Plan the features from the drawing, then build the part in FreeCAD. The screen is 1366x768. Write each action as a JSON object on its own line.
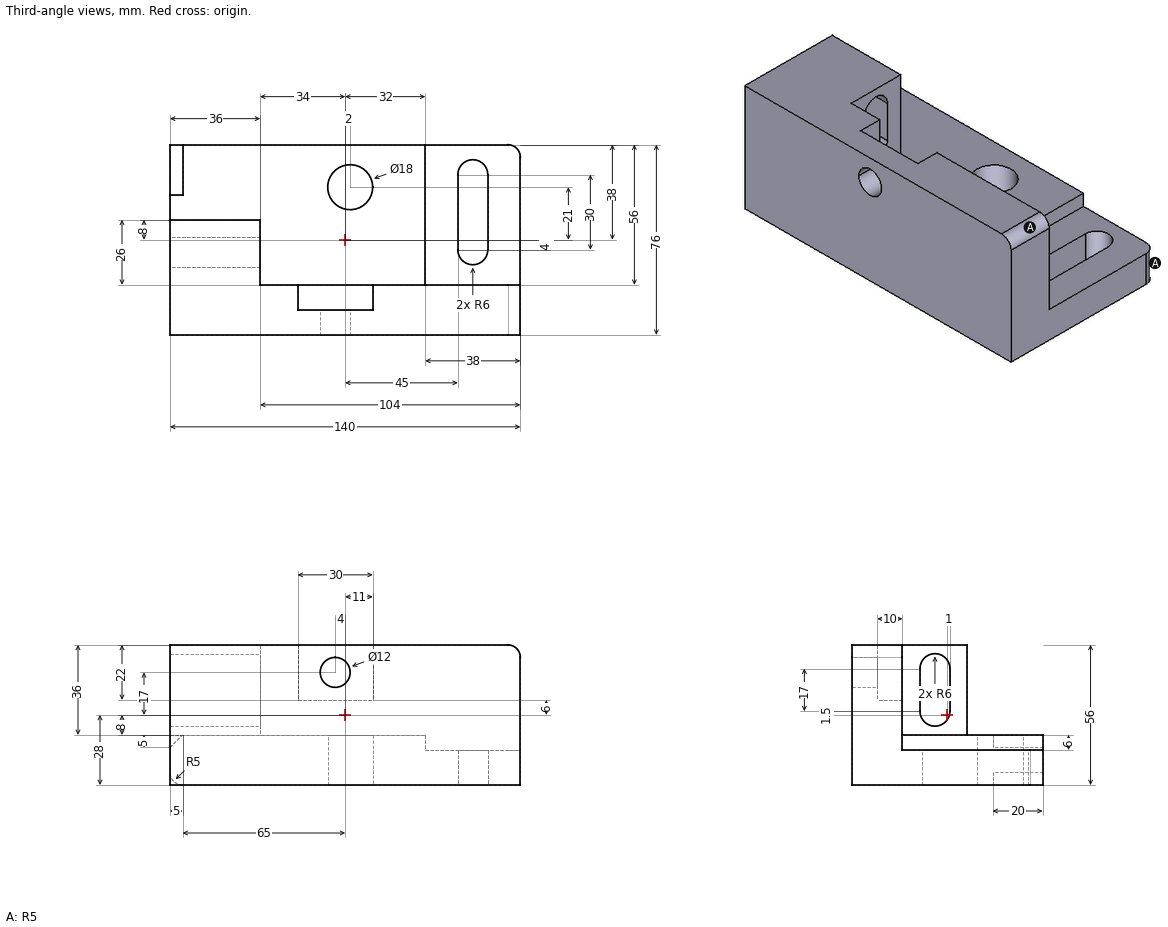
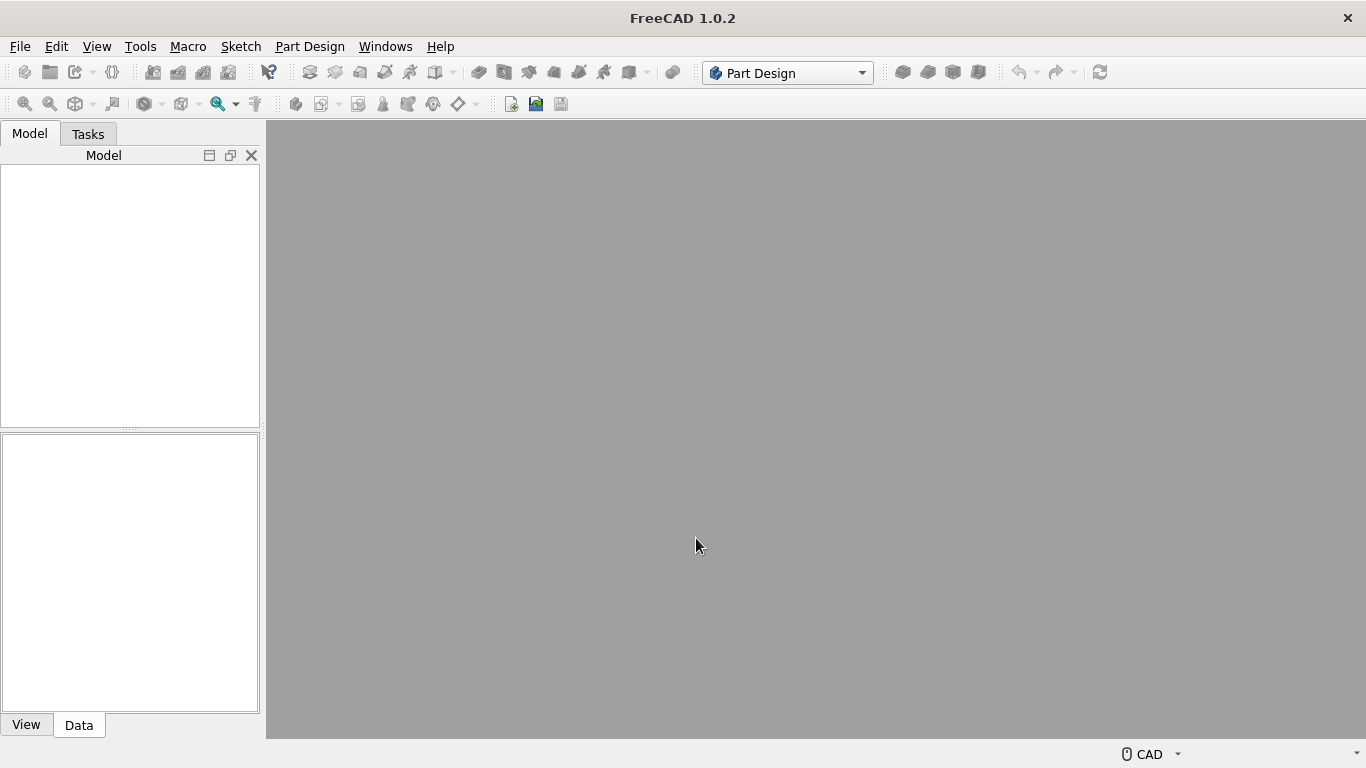
{"action": "key", "text": "ctrl+n"}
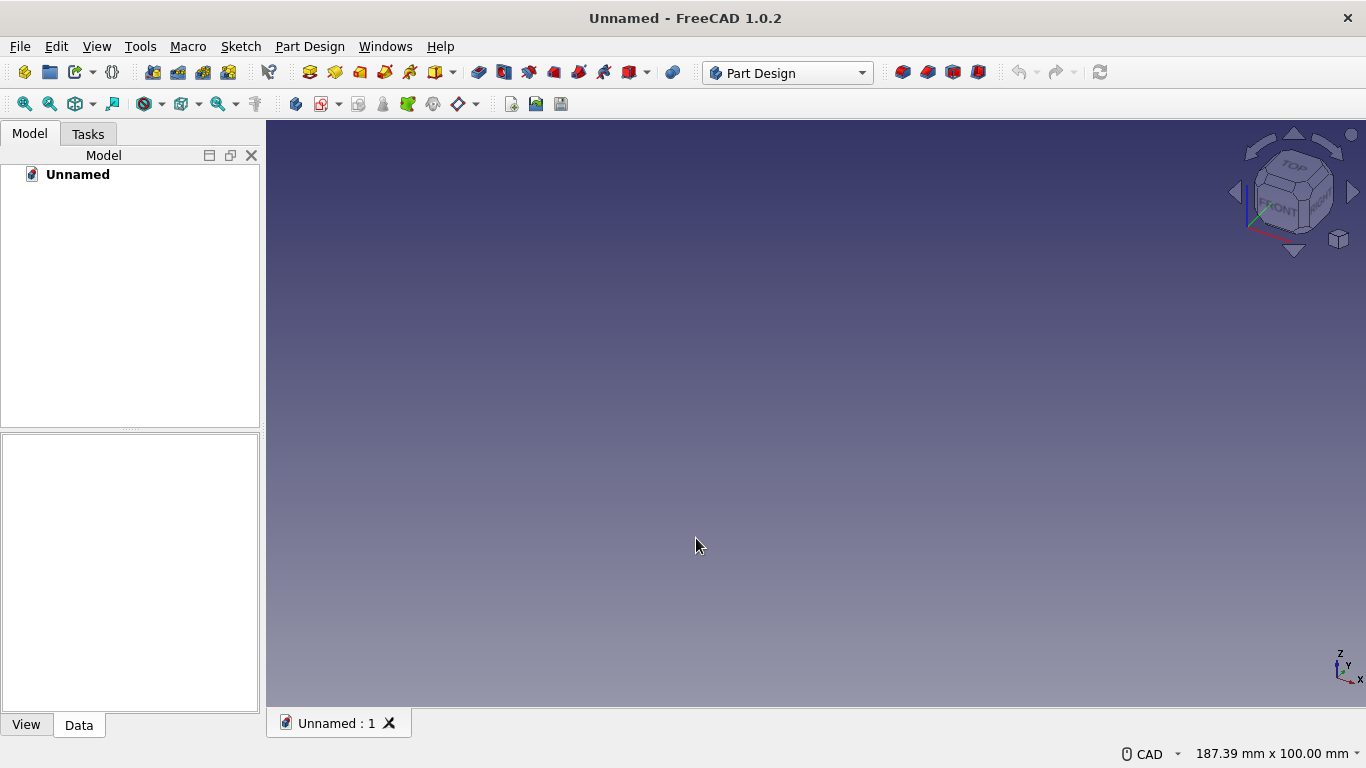
{"action": "left_click", "coordinate": [320, 104]}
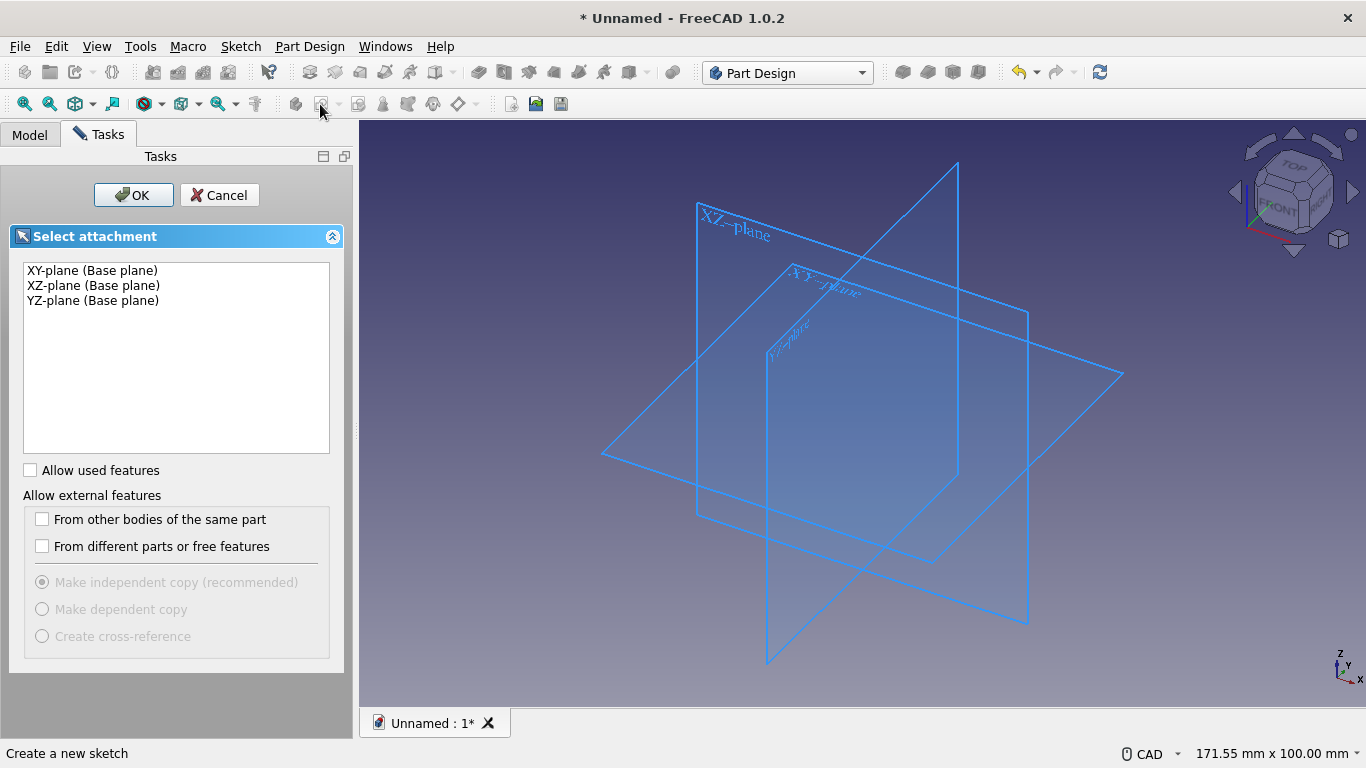
{"action": "left_click", "coordinate": [84, 270]}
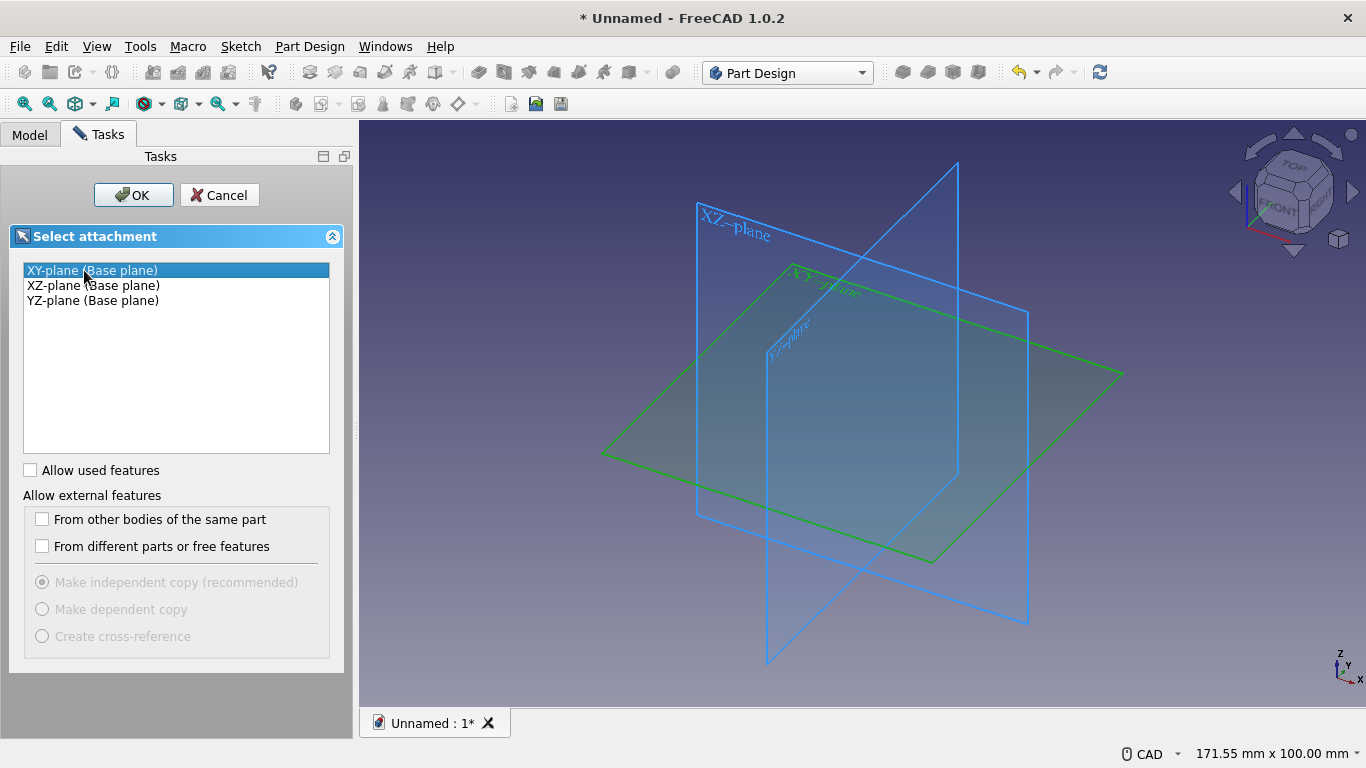
{"action": "left_click", "coordinate": [134, 195]}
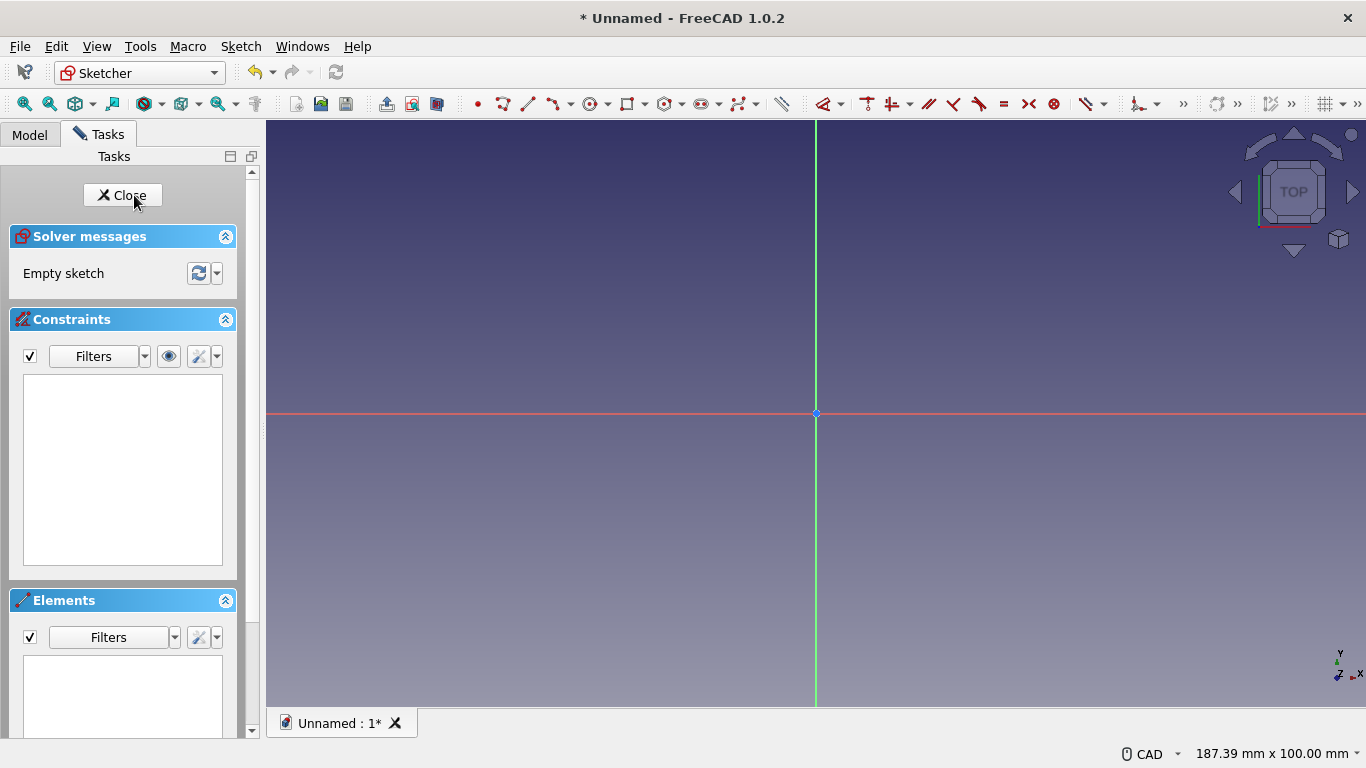
{"action": "scroll", "coordinate": [438, 413], "scroll_direction": "down", "scroll_amount": 1}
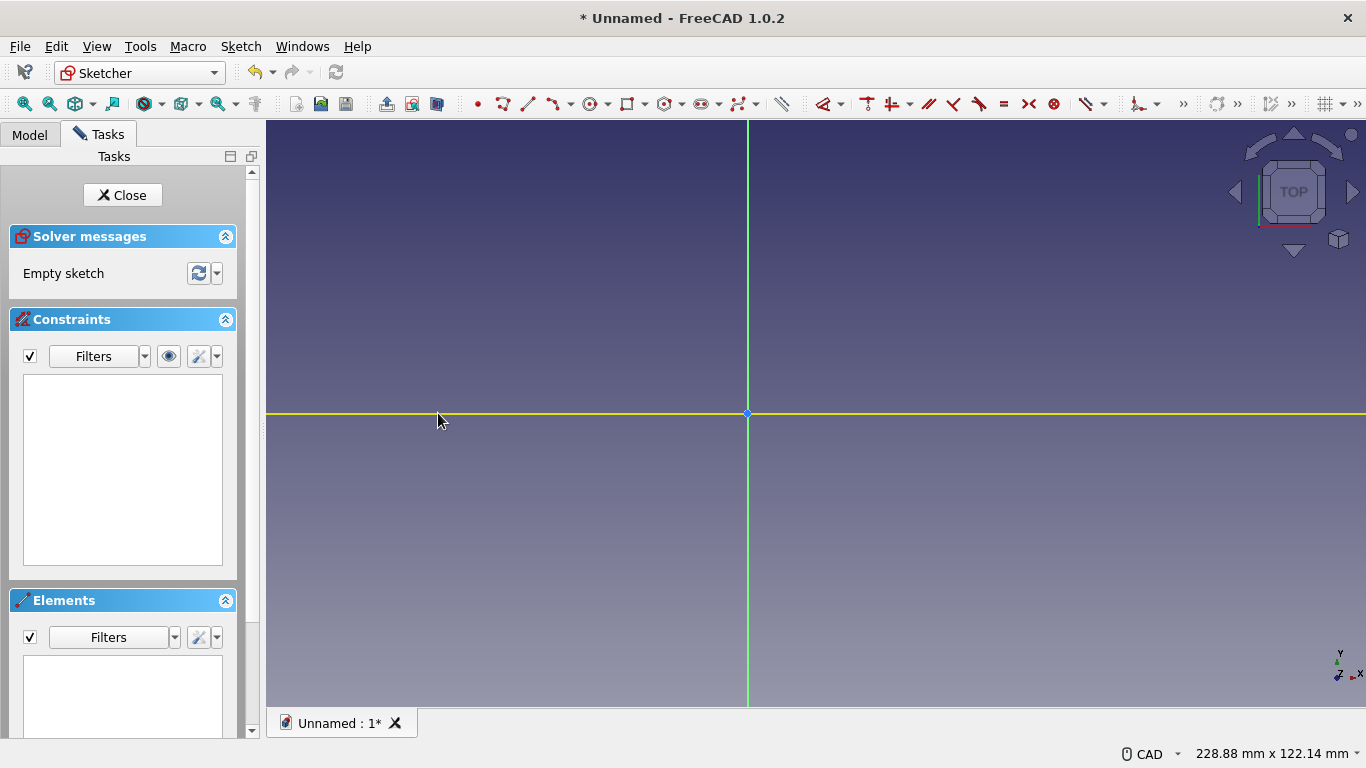
{"action": "key", "text": "g v"}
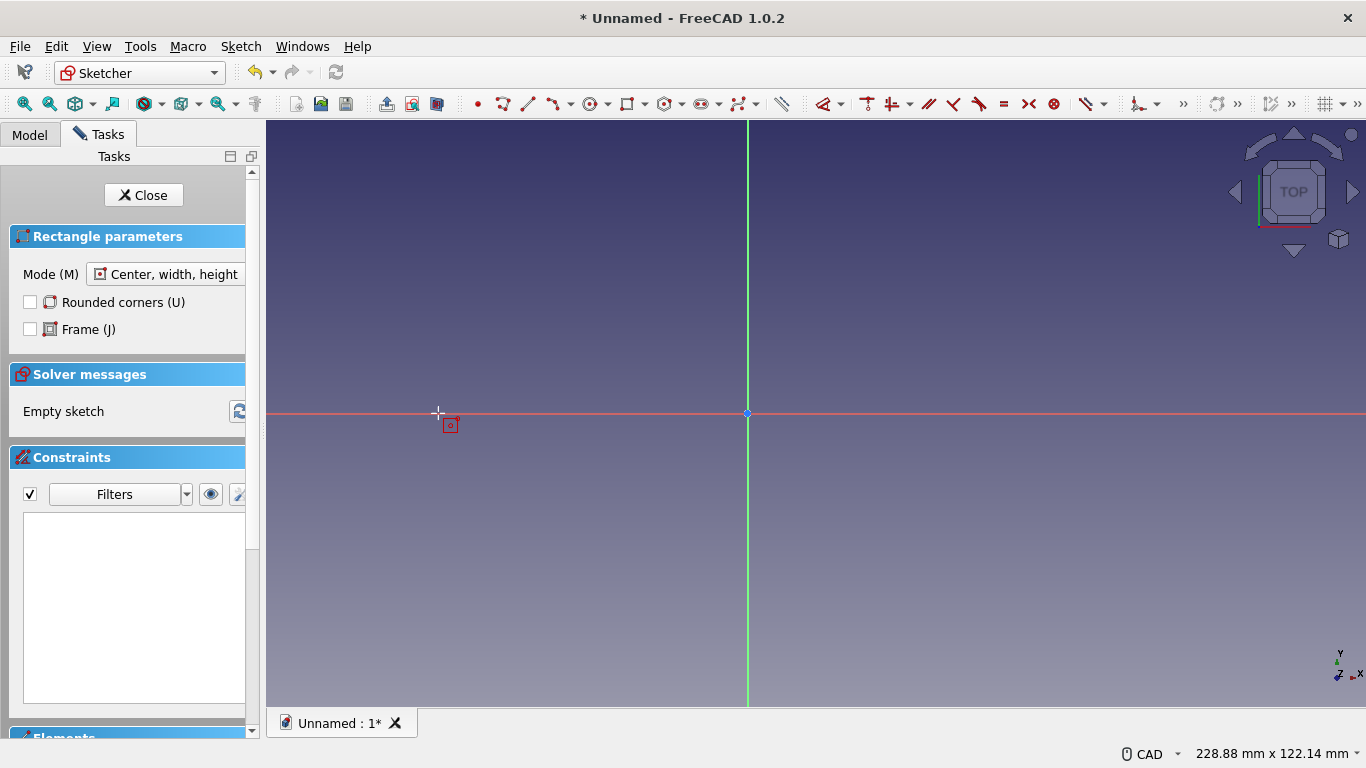
{"action": "left_click", "coordinate": [748, 414]}
{"action": "mouse_move", "coordinate": [1084, 231]}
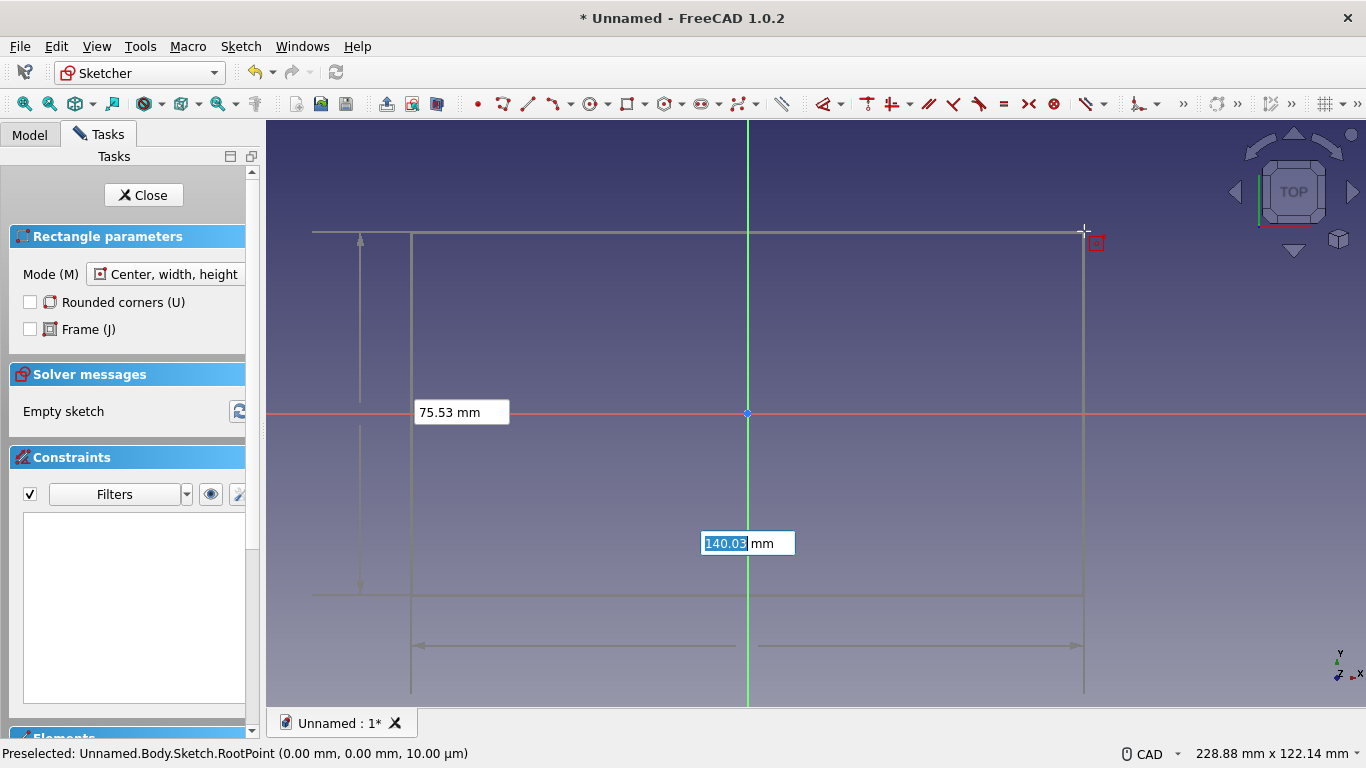
{"action": "type", "text": "140"}
{"action": "key", "text": "Tab"}
{"action": "type", "text": "76"}
{"action": "key", "text": "Return"}
{"action": "key", "text": "Escape"}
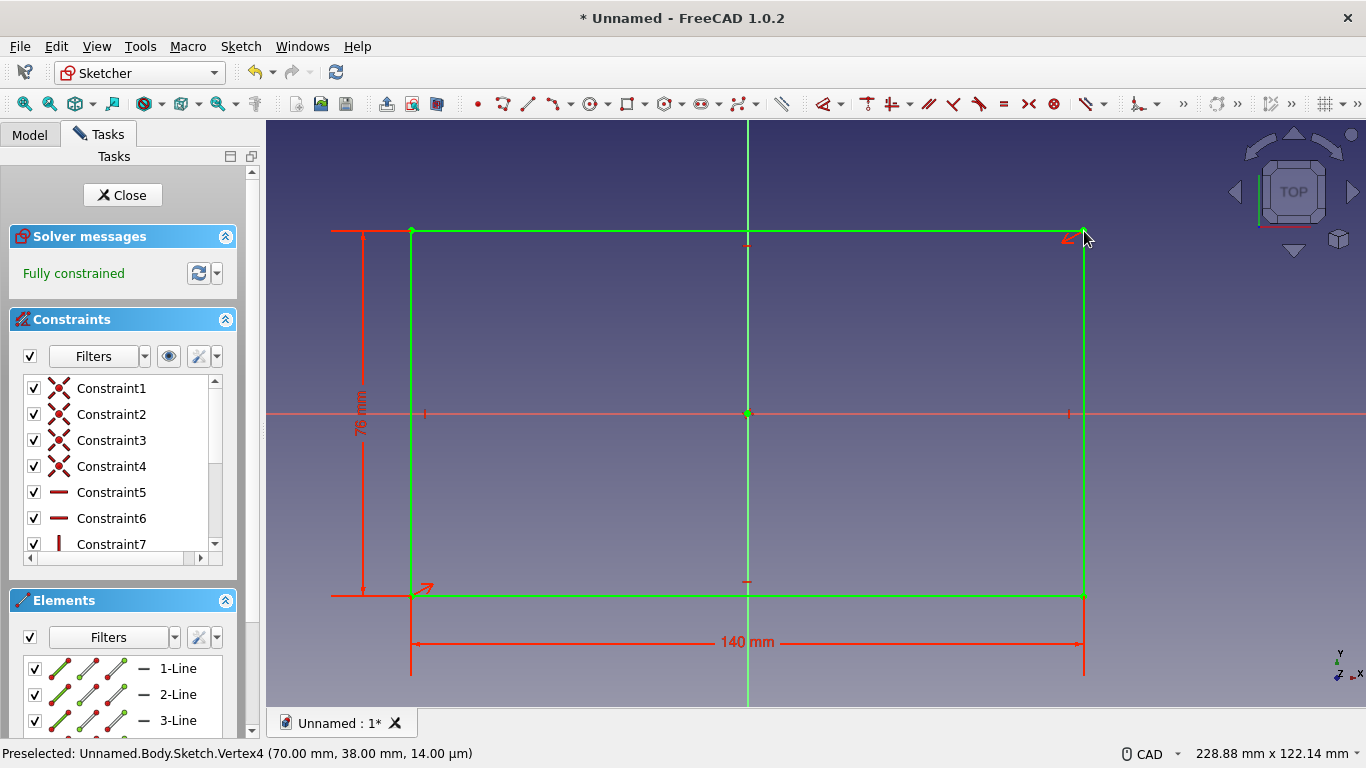
{"action": "left_click", "coordinate": [123, 195]}